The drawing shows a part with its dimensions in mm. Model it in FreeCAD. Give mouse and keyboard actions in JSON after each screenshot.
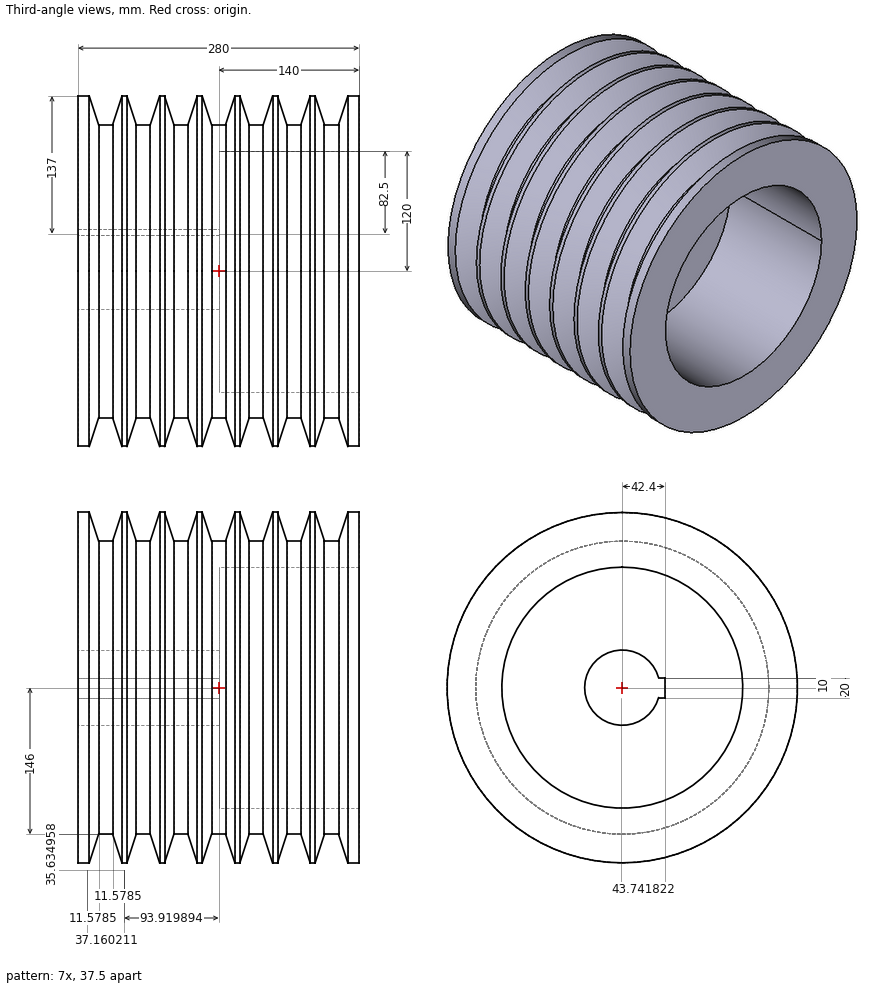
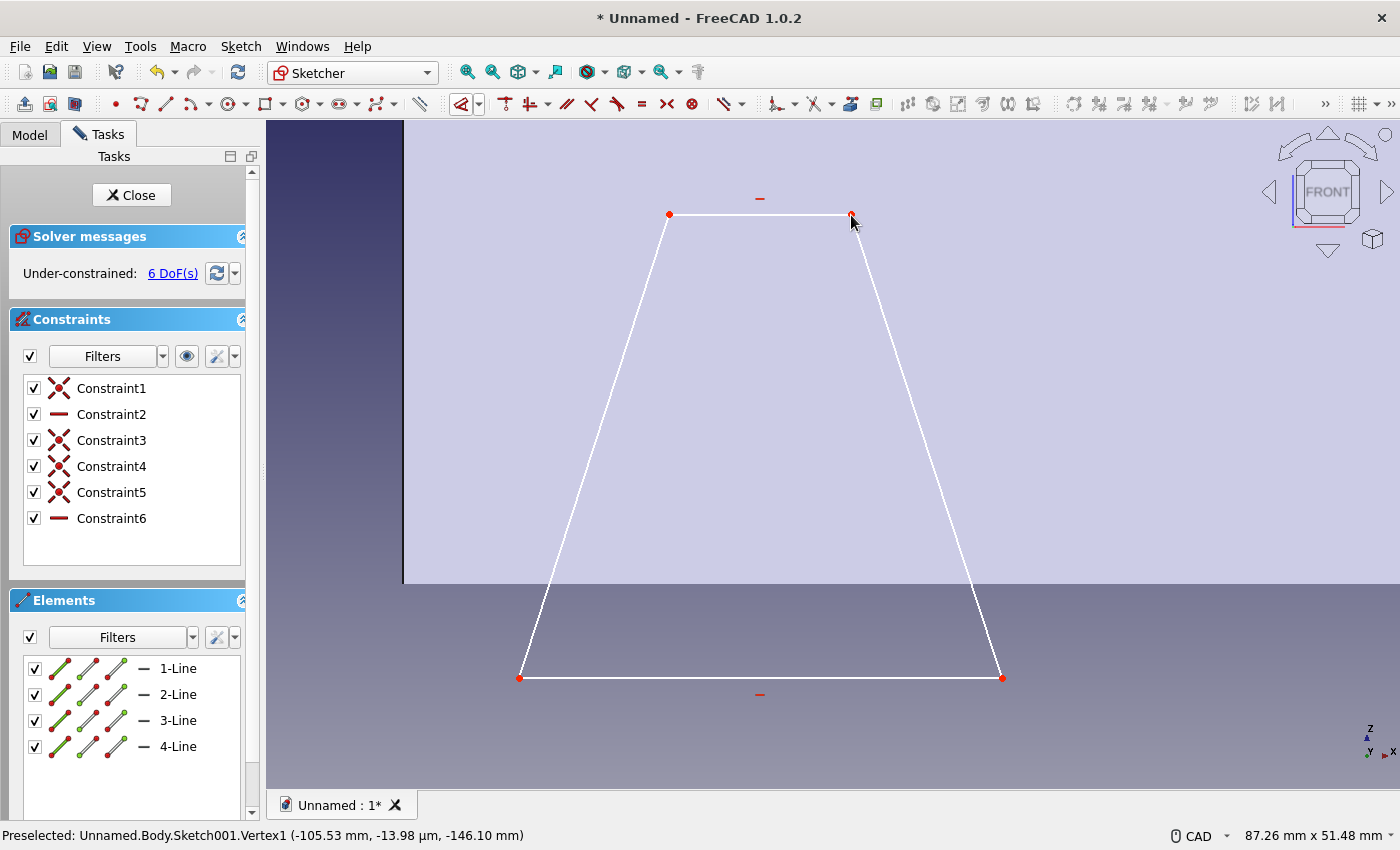
{"action": "left_click", "coordinate": [851, 215]}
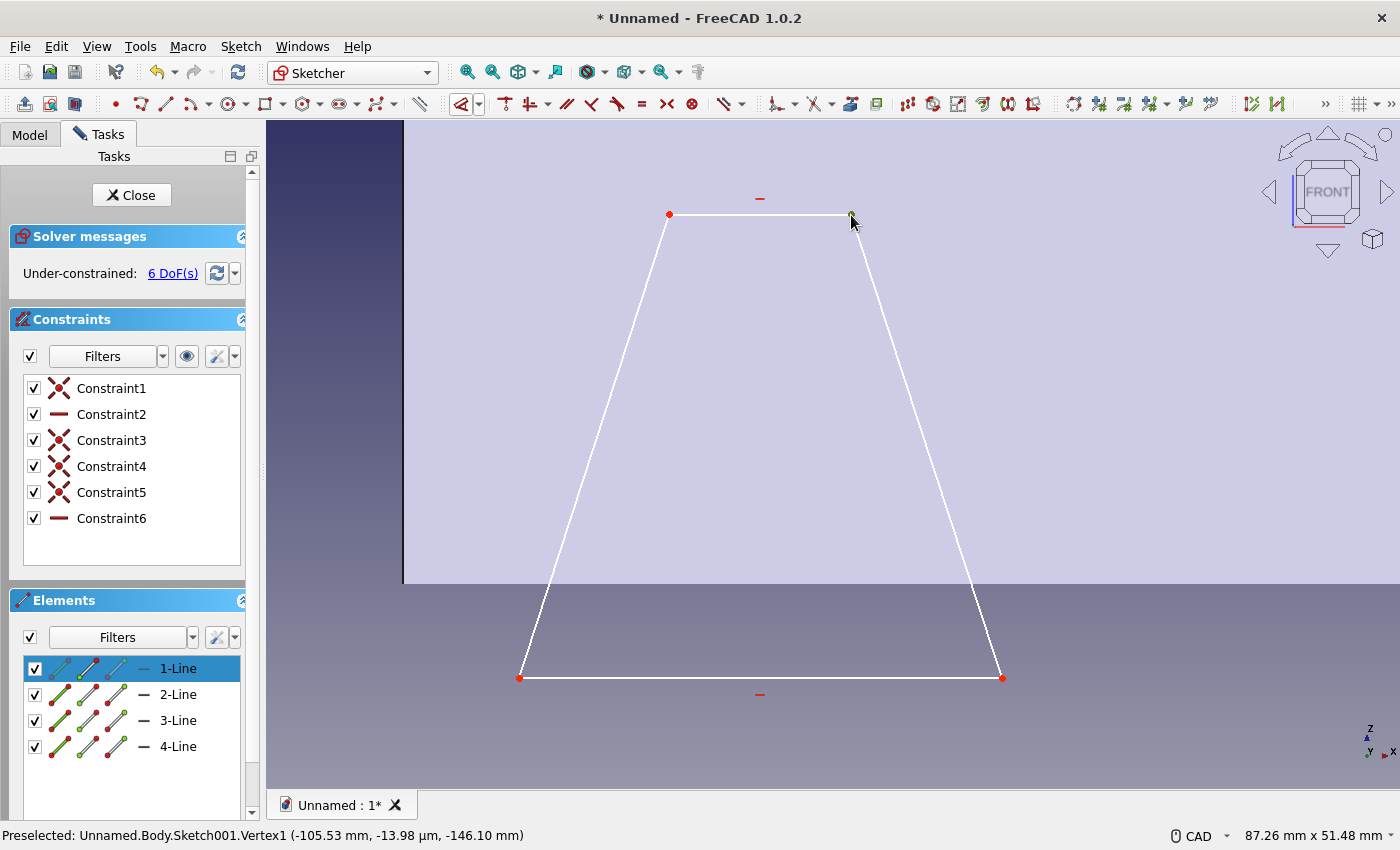
{"action": "key", "text": "i"}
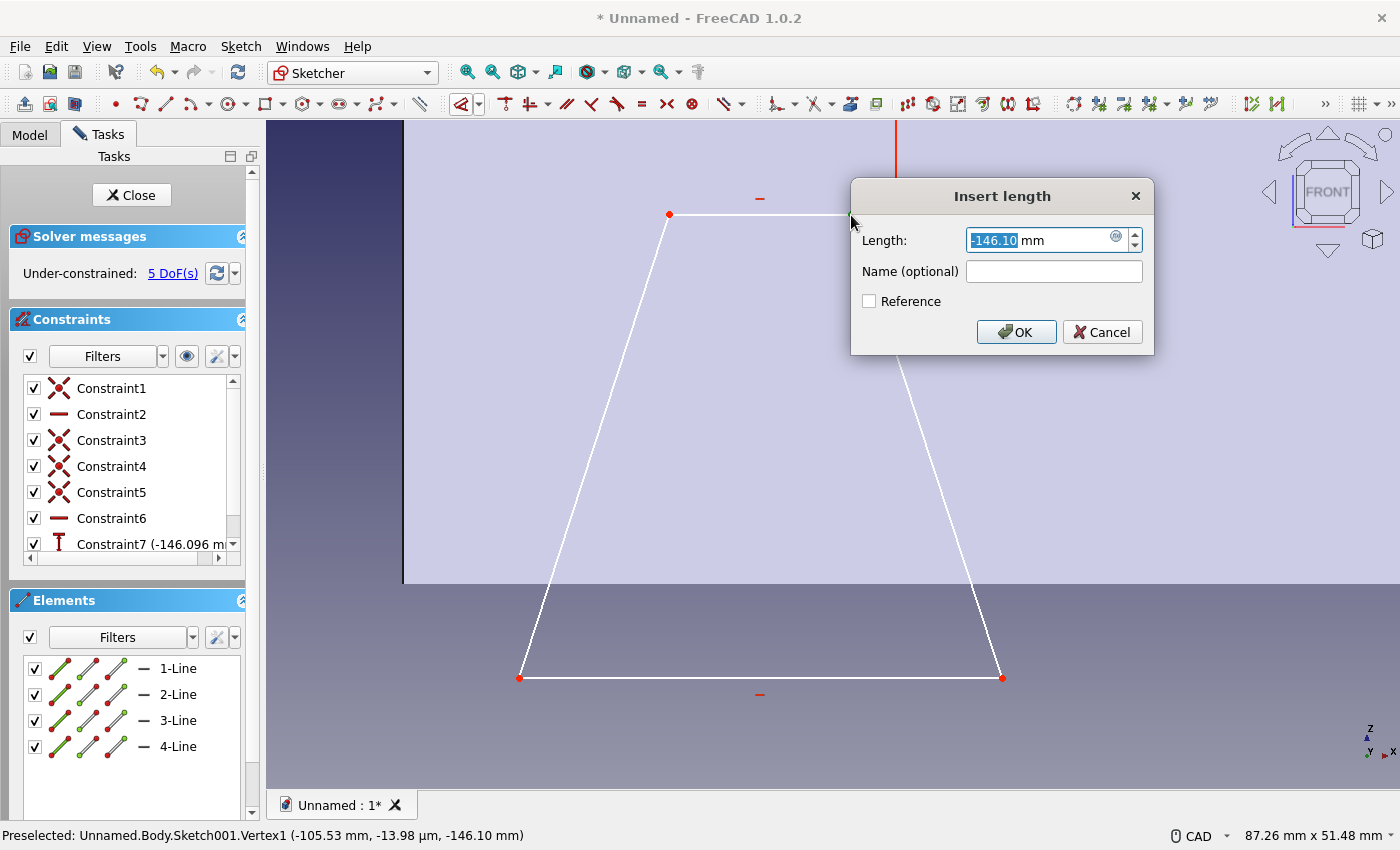
{"action": "type", "text": "-146"}
{"action": "key", "text": "Return"}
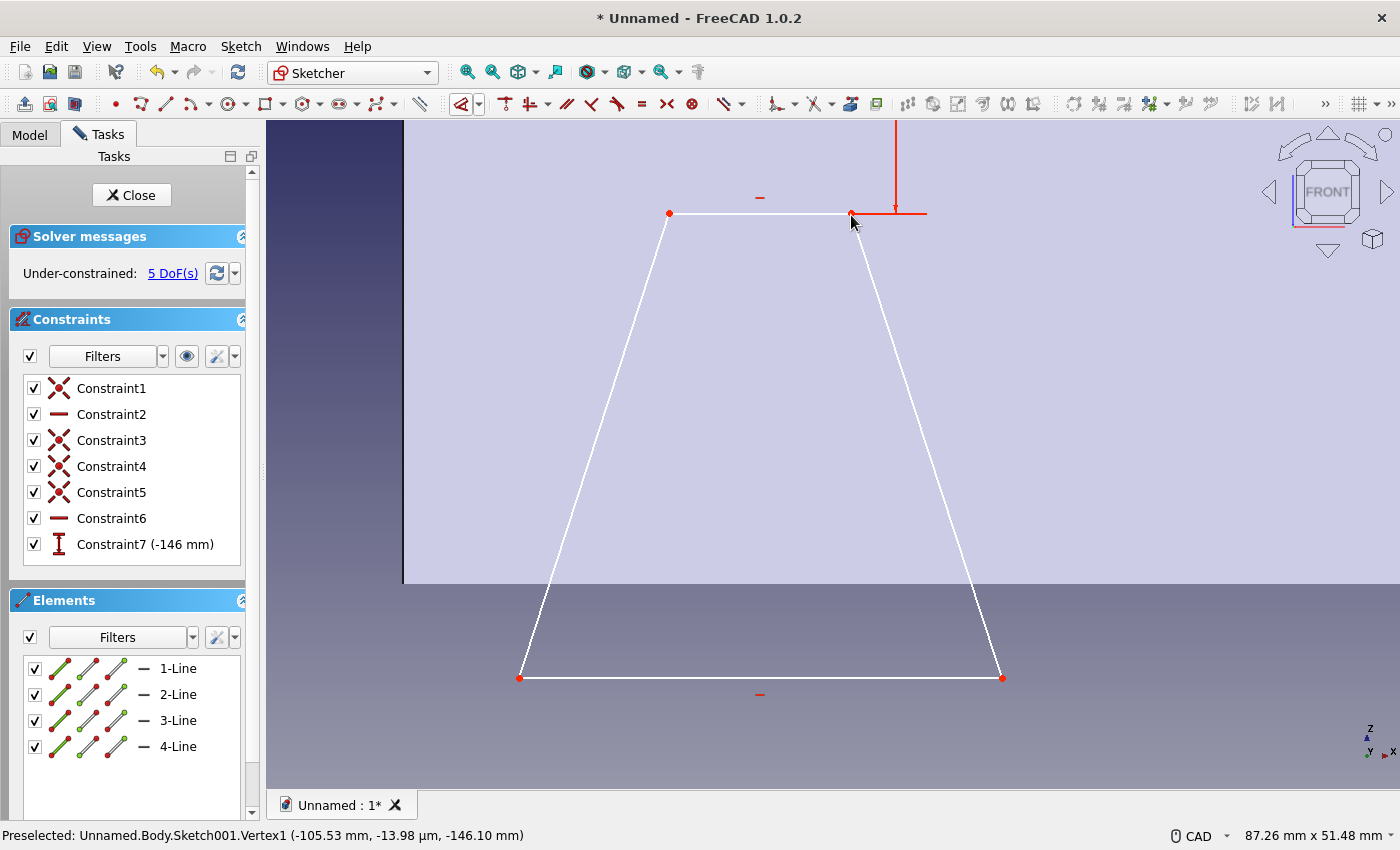
{"action": "left_click", "coordinate": [896, 353]}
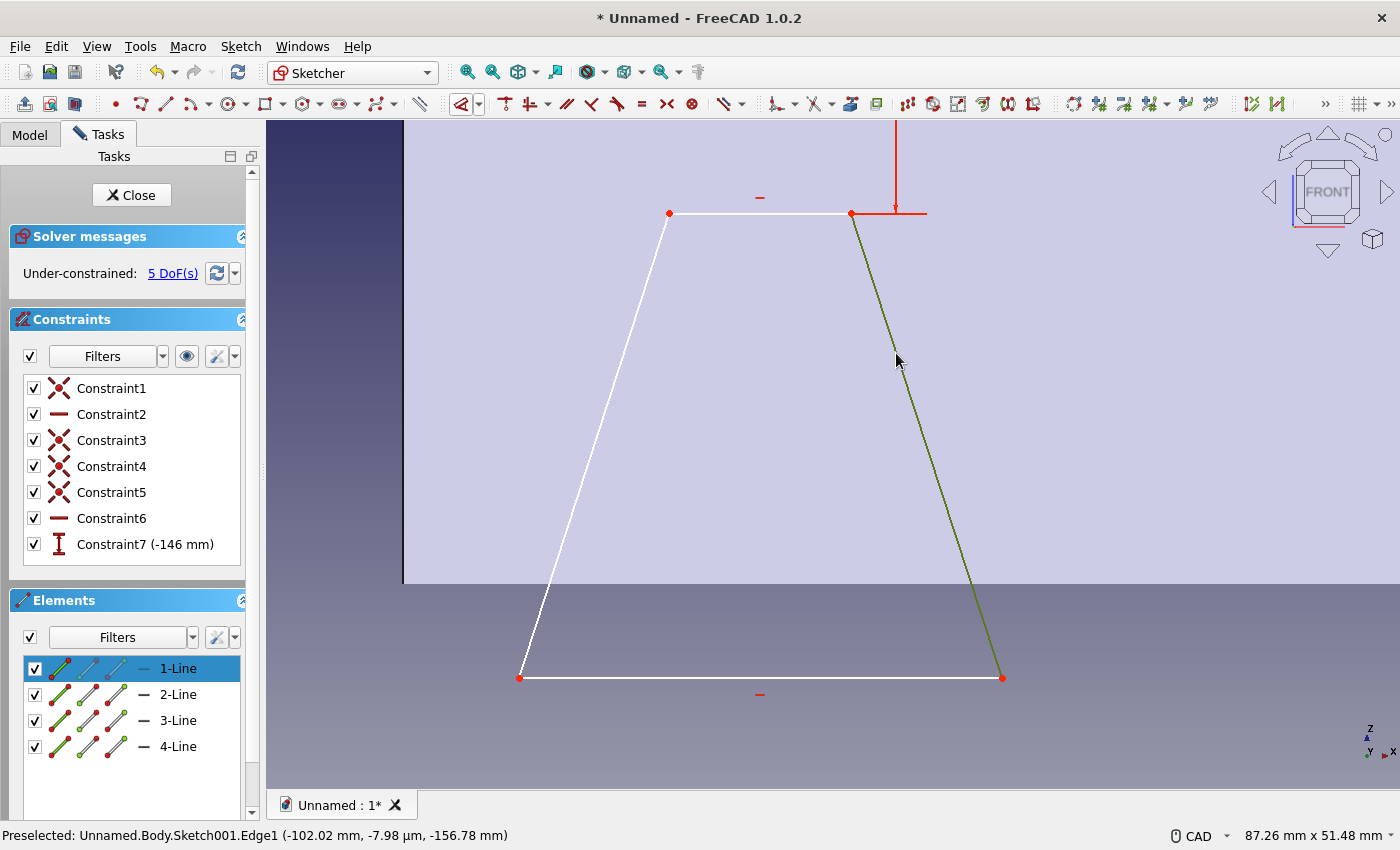
{"action": "left_click", "coordinate": [478, 104]}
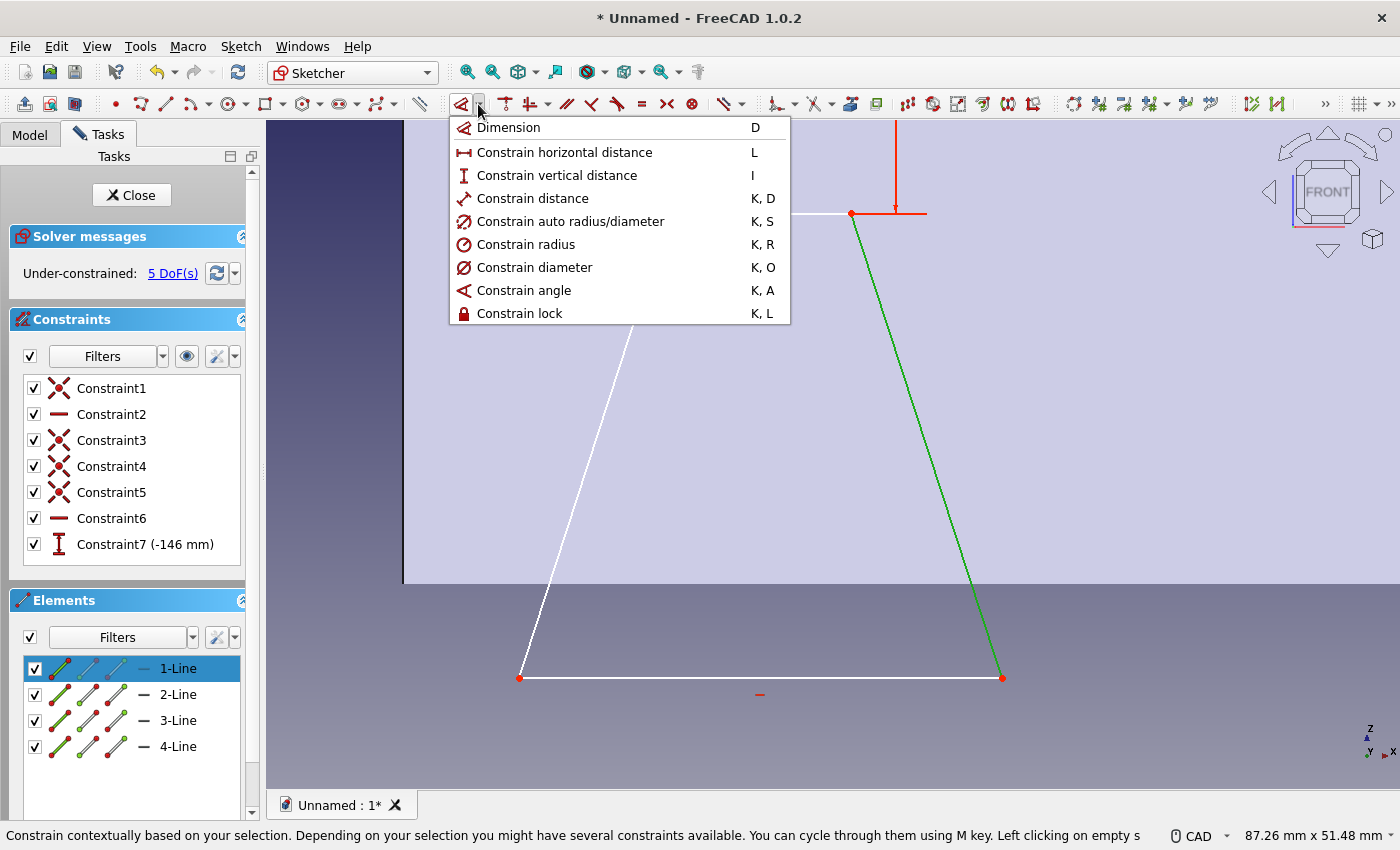
{"action": "left_click", "coordinate": [620, 152]}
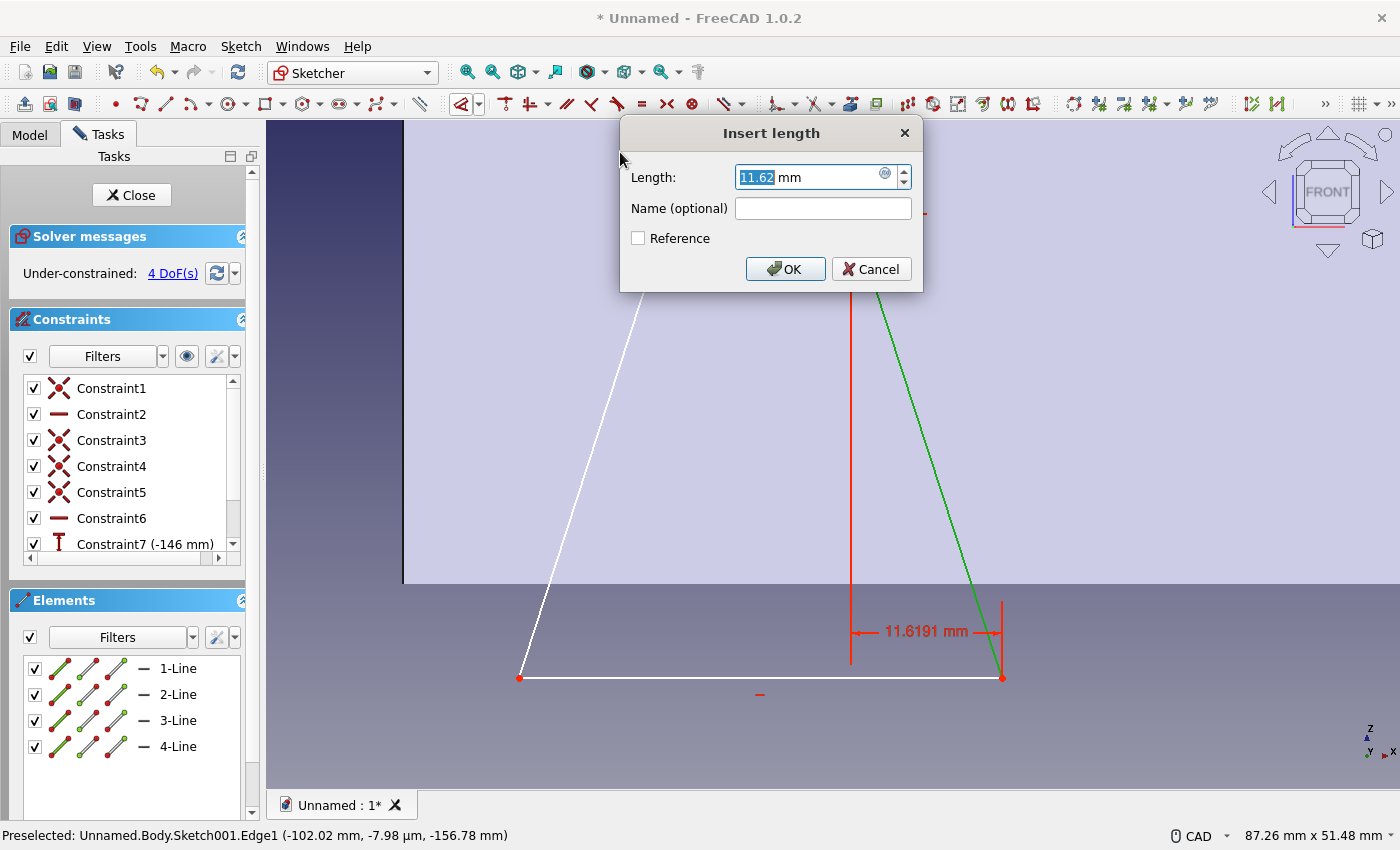
{"action": "type", "text": "11.5785"}
{"action": "key", "text": "Return"}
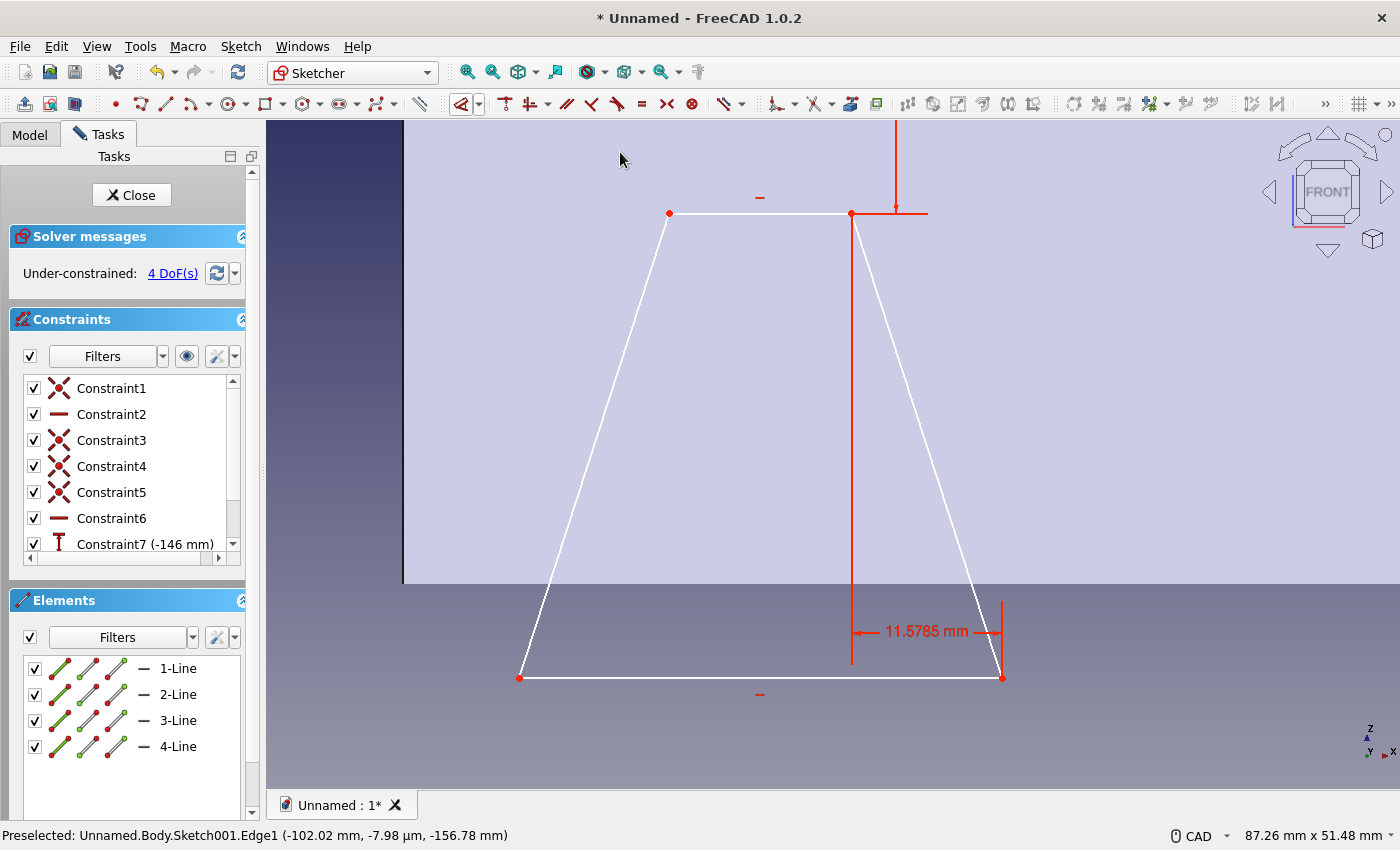
{"action": "left_click", "coordinate": [564, 539]}